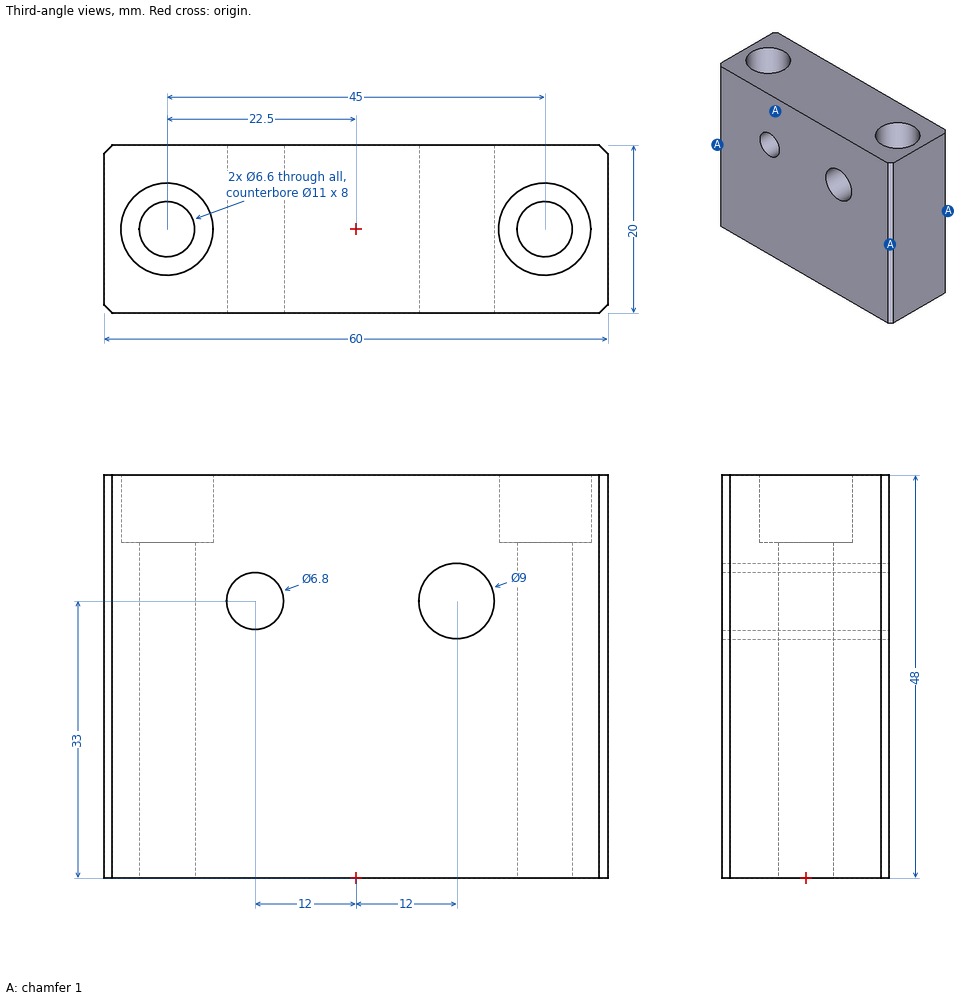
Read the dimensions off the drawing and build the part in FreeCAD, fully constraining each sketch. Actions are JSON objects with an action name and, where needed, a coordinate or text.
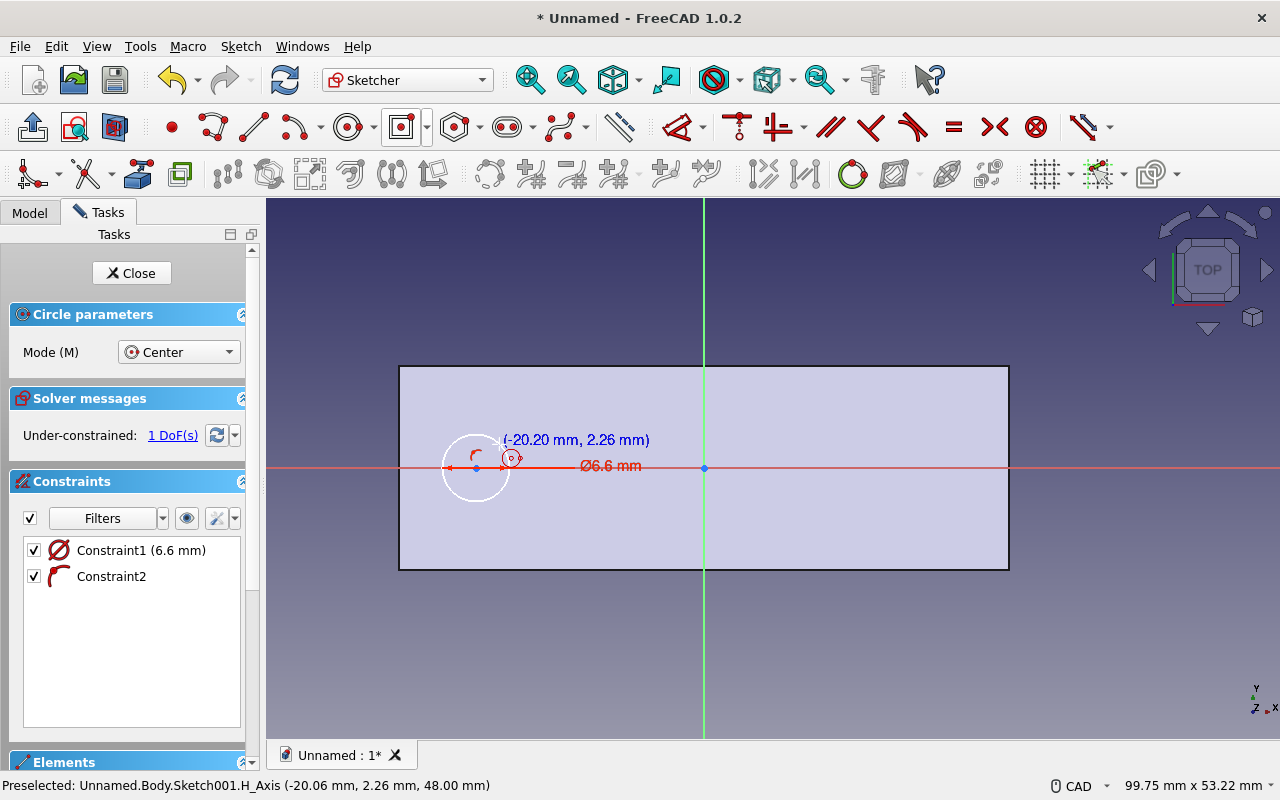
{"action": "left_click", "coordinate": [933, 468]}
{"action": "mouse_move", "coordinate": [957, 444]}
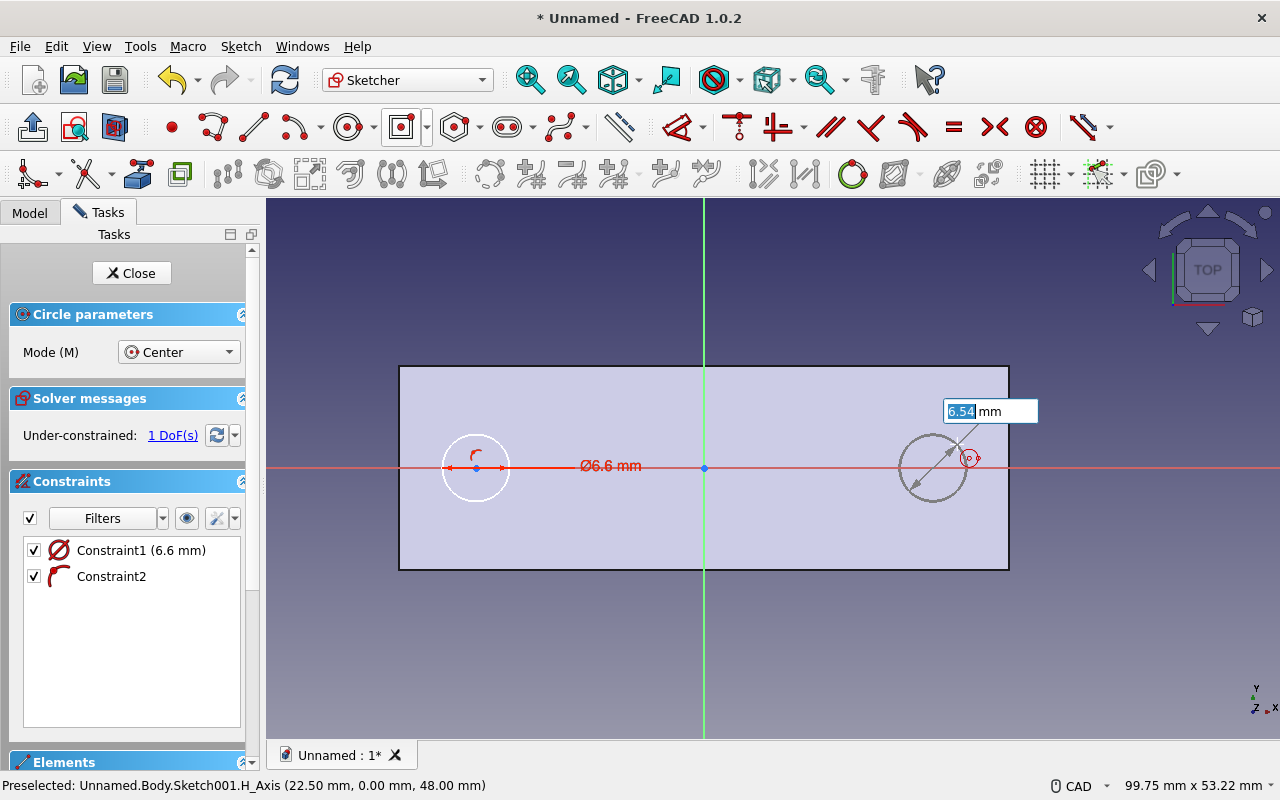
{"action": "type", "text": "6.6"}
{"action": "key", "text": "Return"}
{"action": "key", "text": "Escape"}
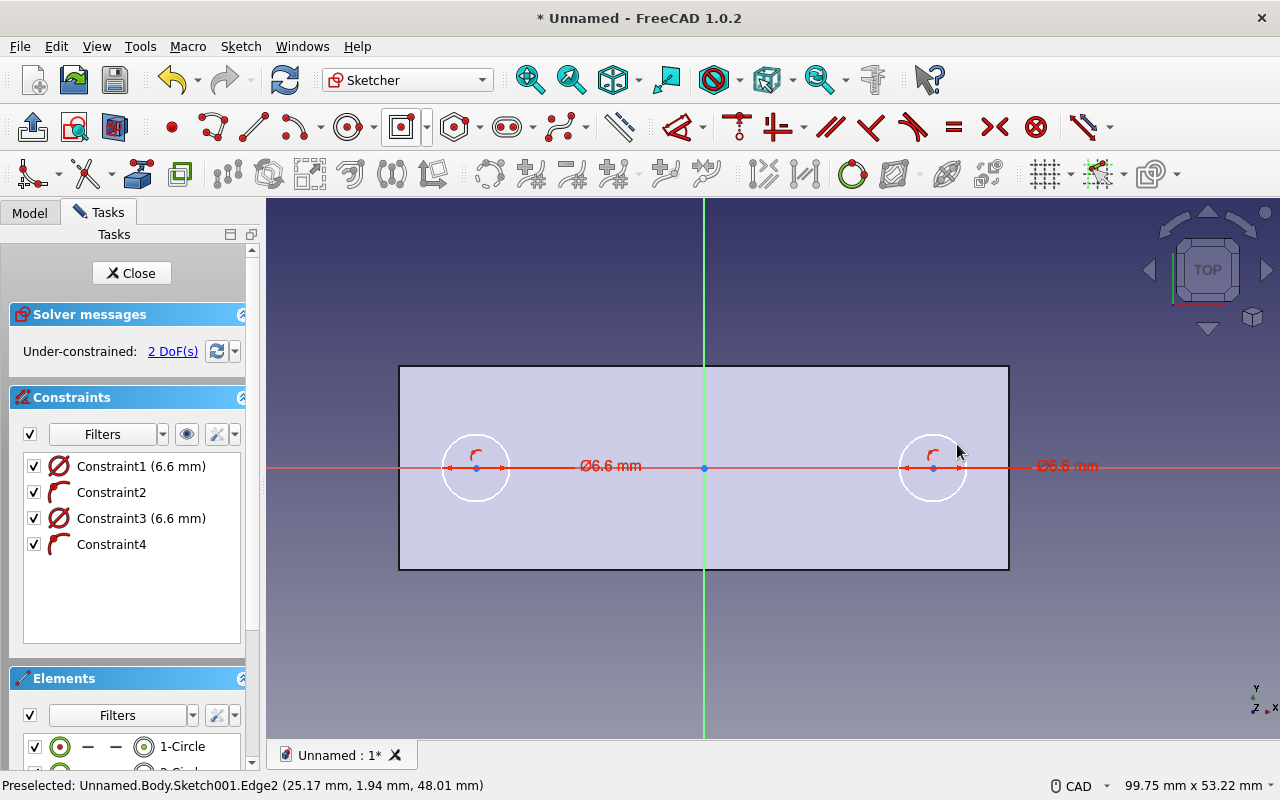
{"action": "left_click", "coordinate": [676, 128]}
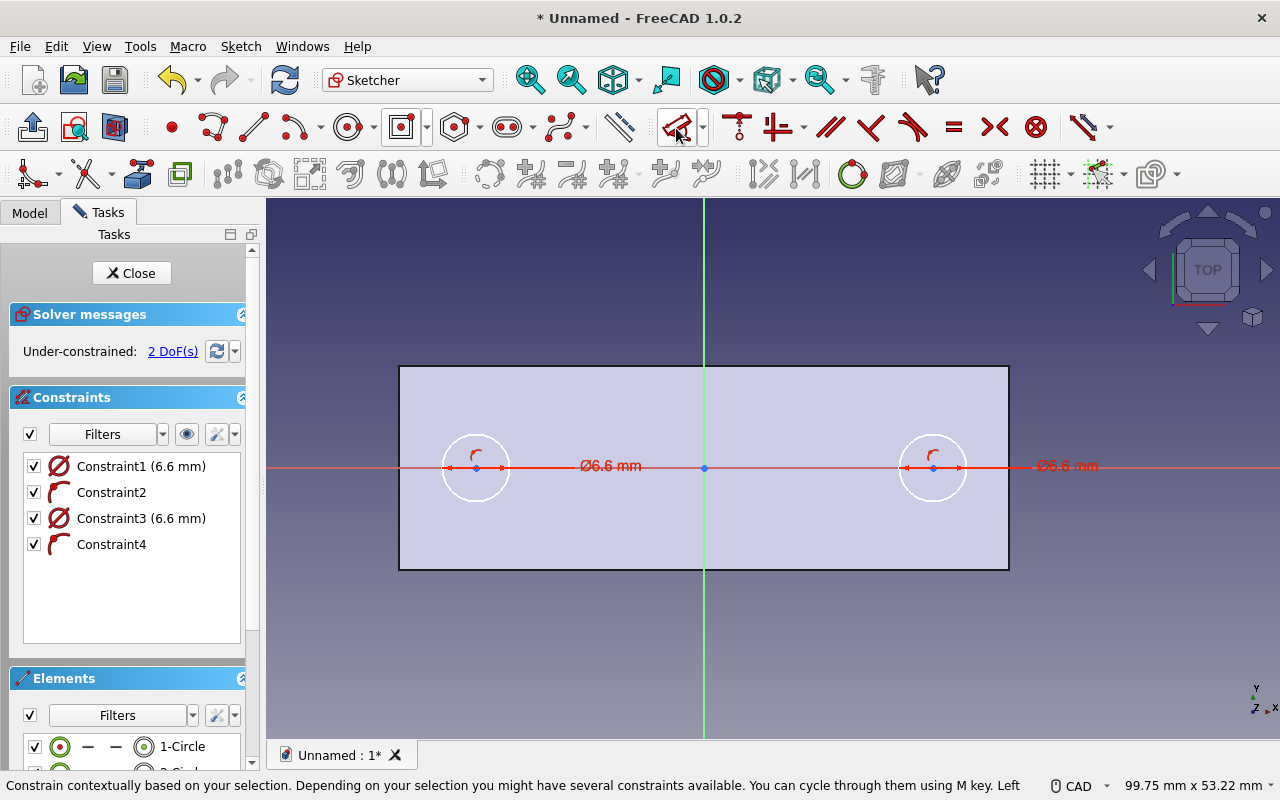
{"action": "left_click", "coordinate": [476, 468]}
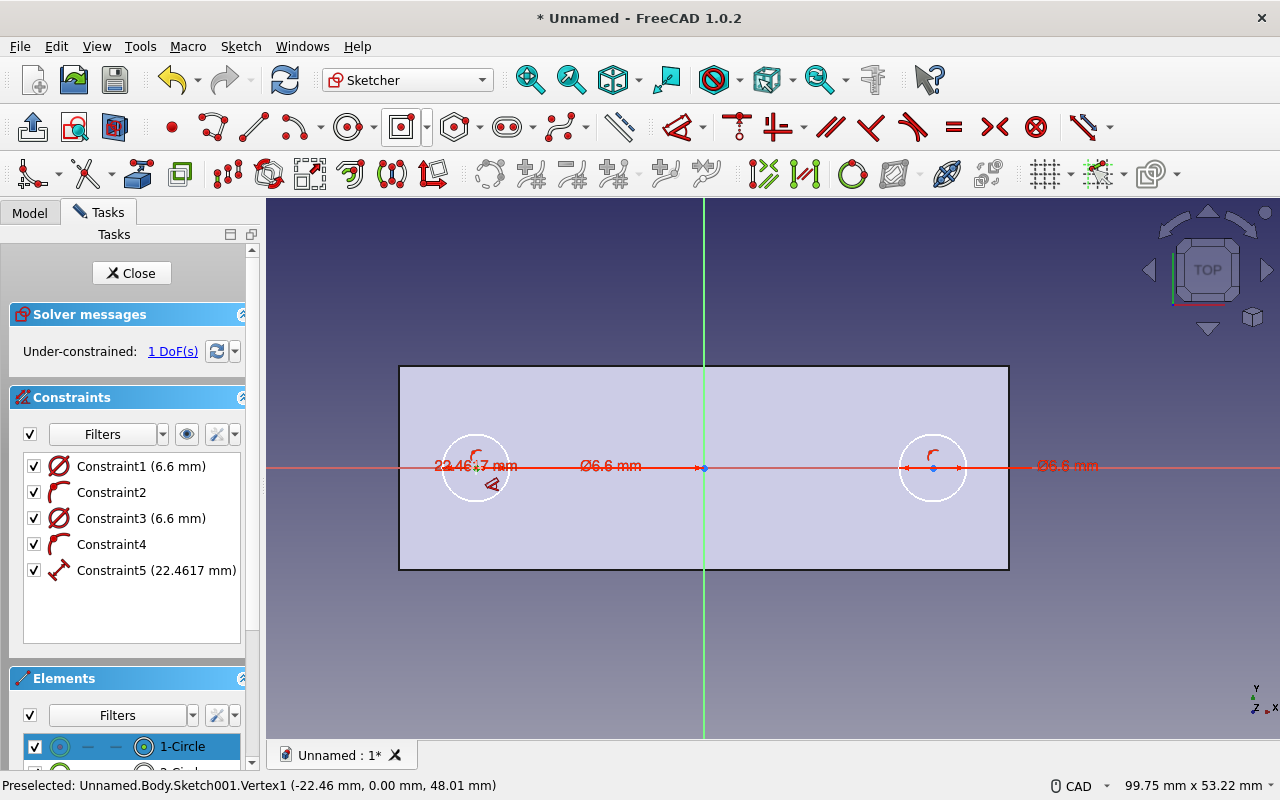
{"action": "left_click", "coordinate": [933, 468]}
{"action": "left_click", "coordinate": [599, 502]}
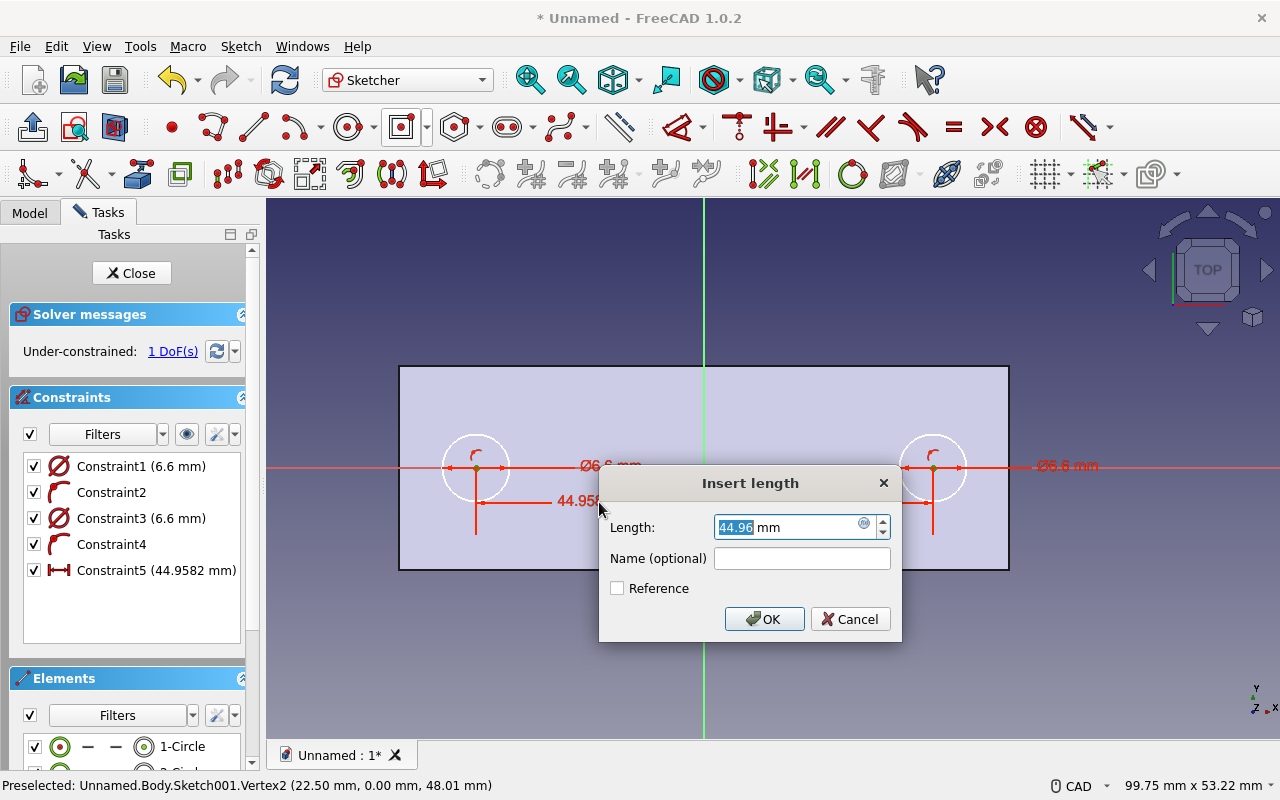
{"action": "type", "text": "45"}
{"action": "key", "text": "Return"}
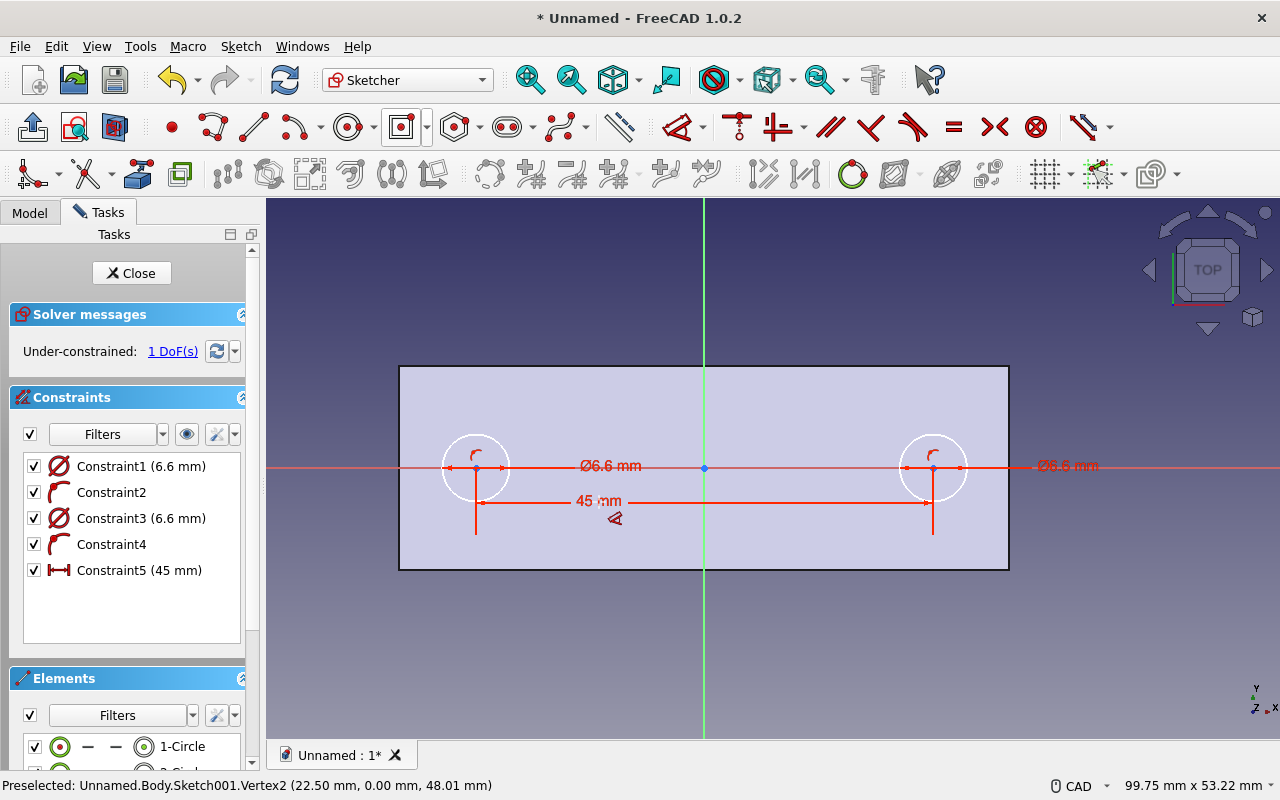
{"action": "left_click", "coordinate": [476, 468]}
{"action": "left_click", "coordinate": [510, 502]}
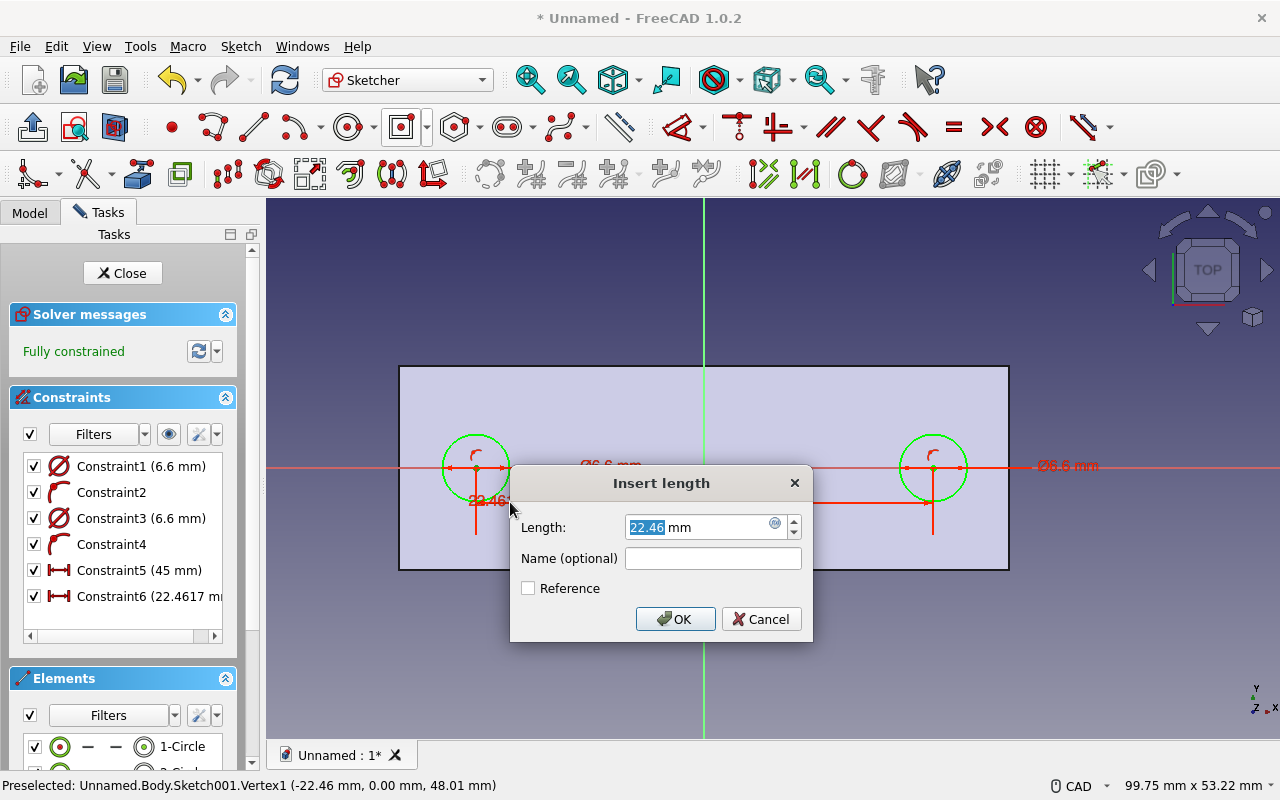
{"action": "type", "text": "22.5"}
{"action": "key", "text": "Return"}
{"action": "key", "text": "Escape"}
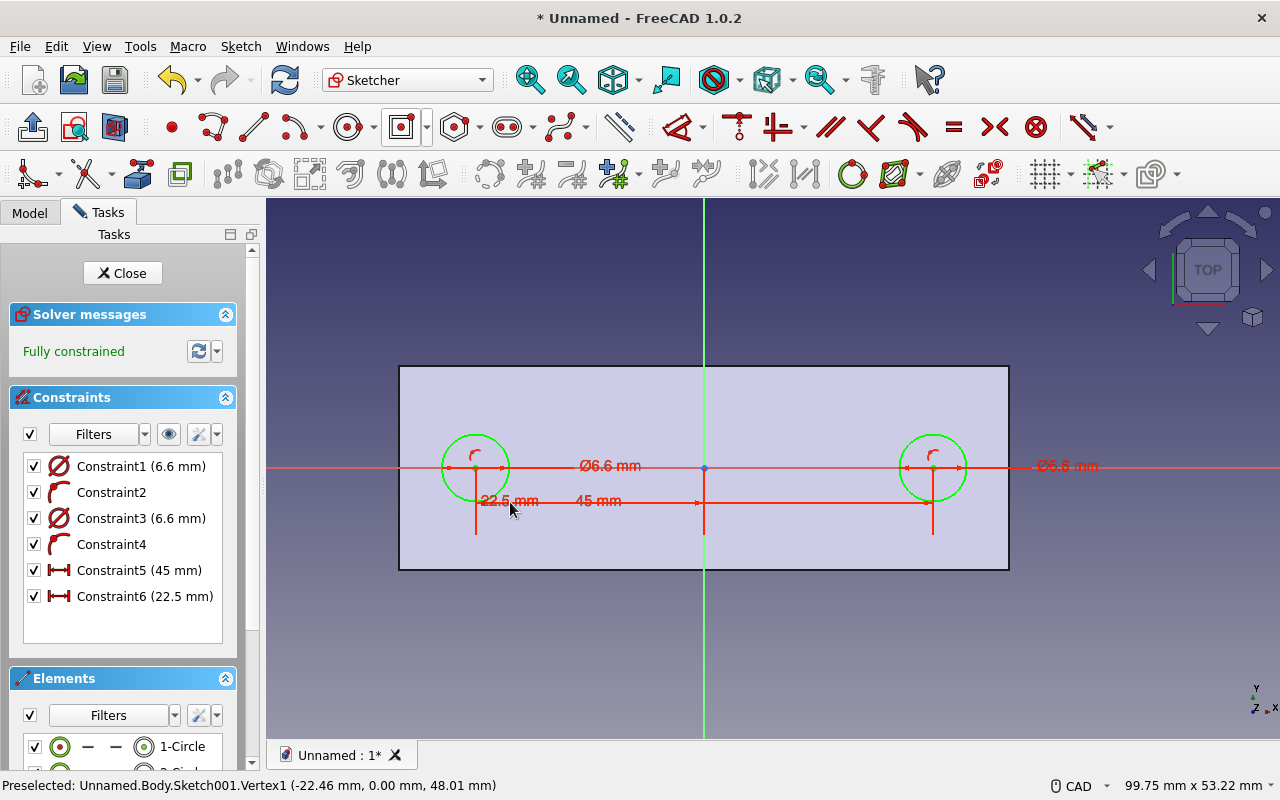
{"action": "left_click", "coordinate": [123, 273]}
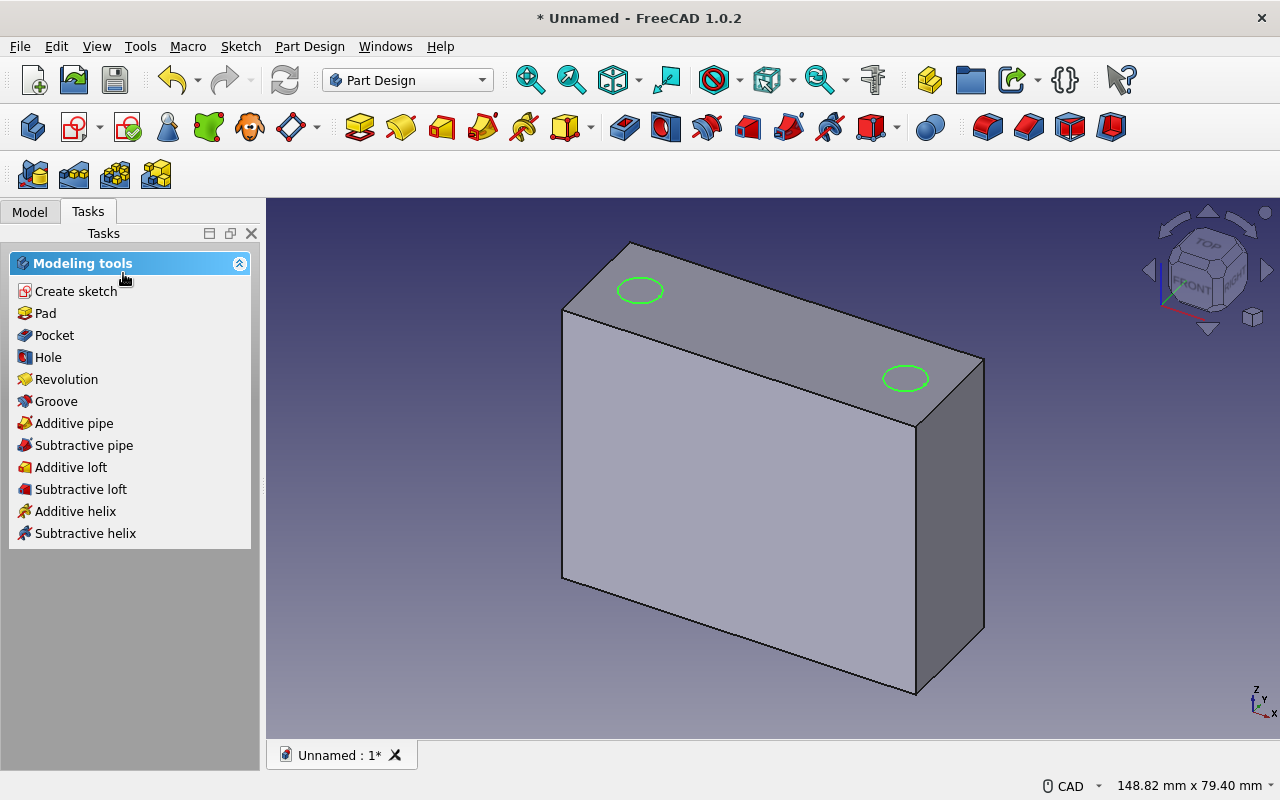
{"action": "left_click", "coordinate": [666, 128]}